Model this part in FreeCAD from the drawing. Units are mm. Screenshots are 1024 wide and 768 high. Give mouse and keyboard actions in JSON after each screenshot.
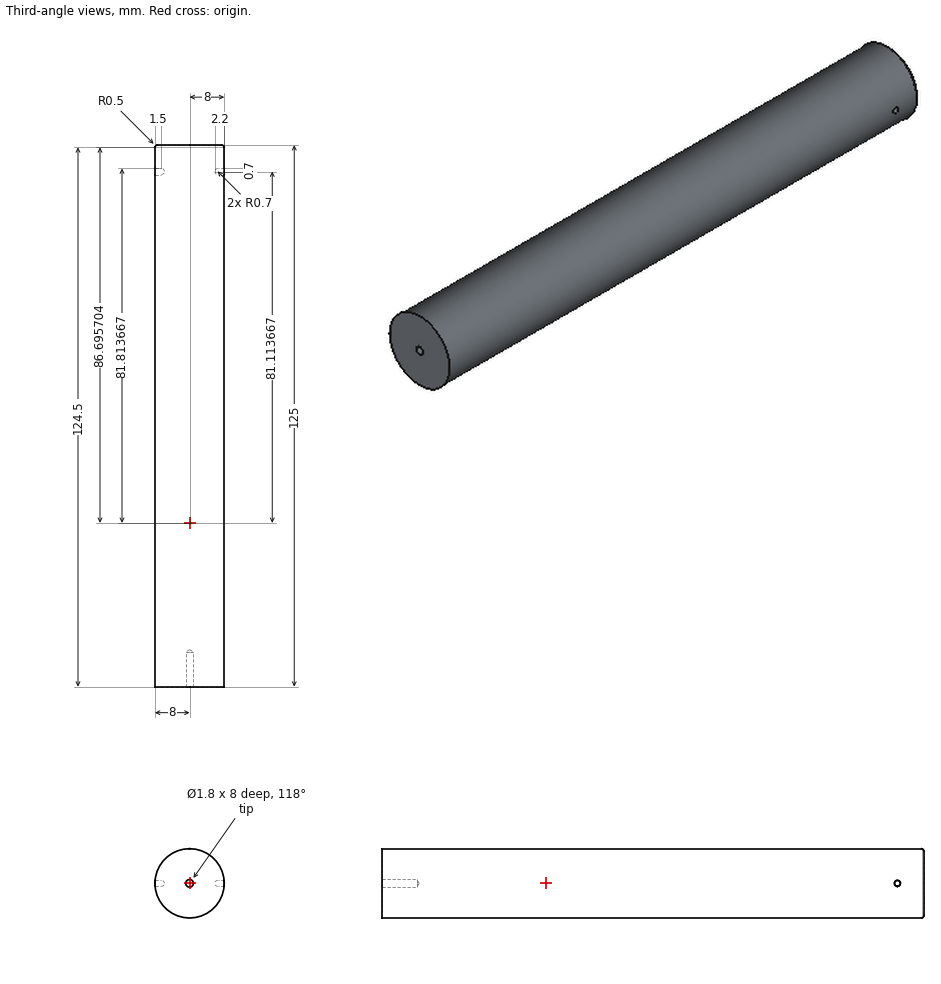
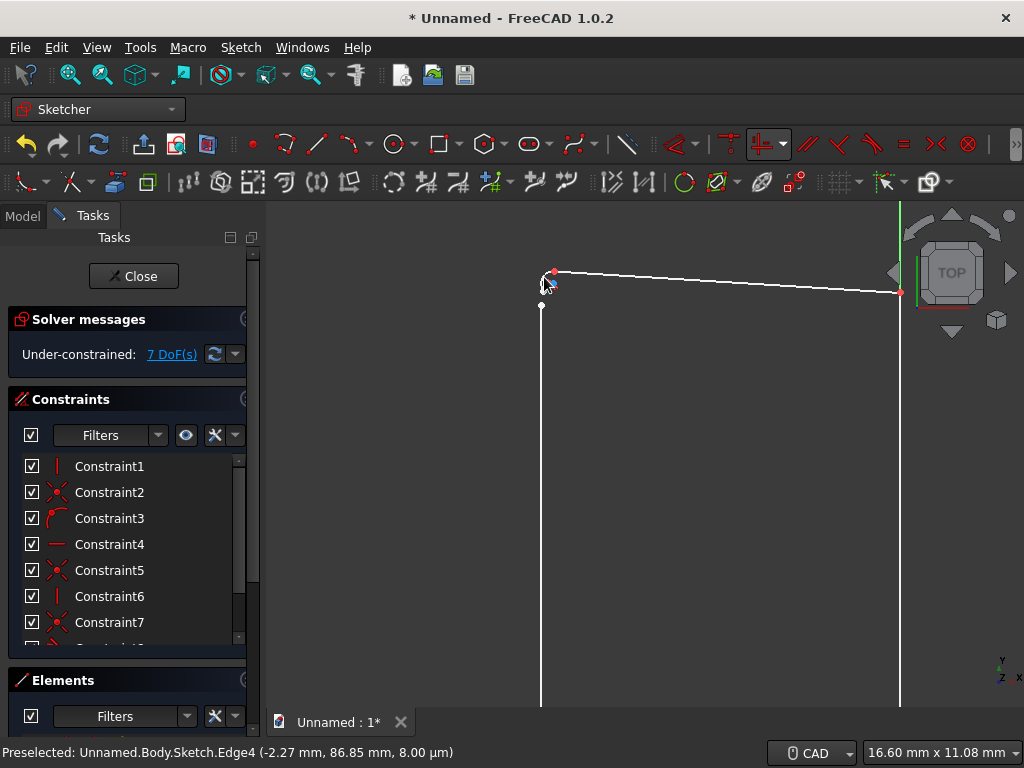
{"action": "scroll", "coordinate": [567, 281], "scroll_direction": "down", "scroll_amount": 14}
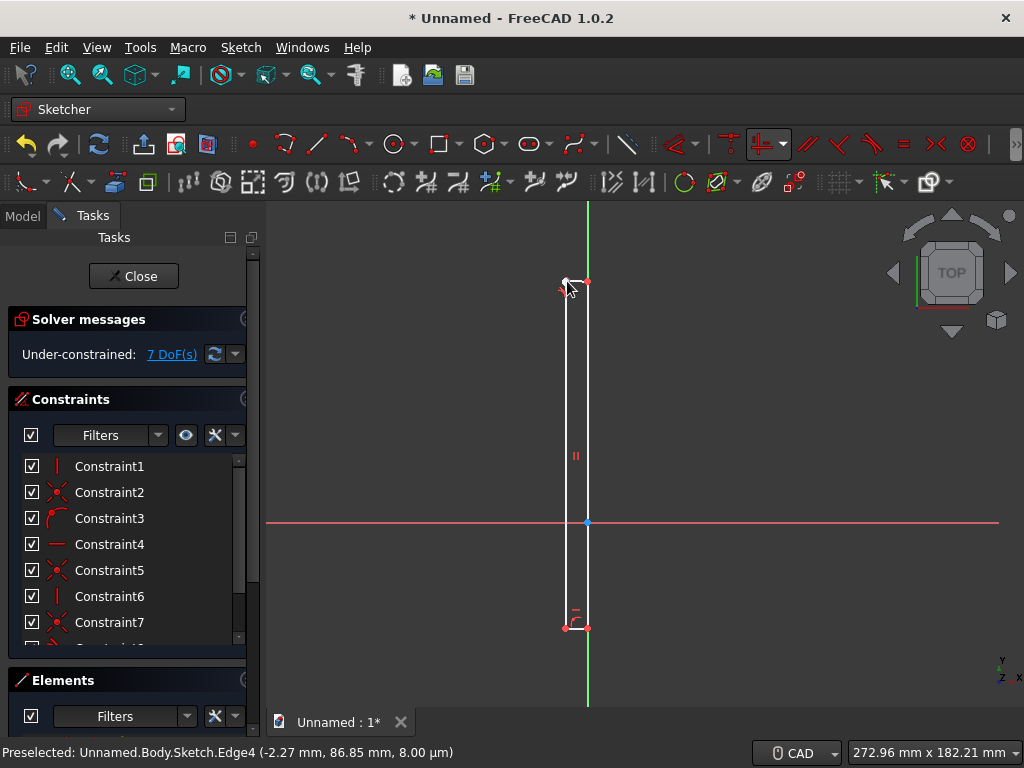
{"action": "scroll", "coordinate": [581, 281], "scroll_direction": "up", "scroll_amount": 4}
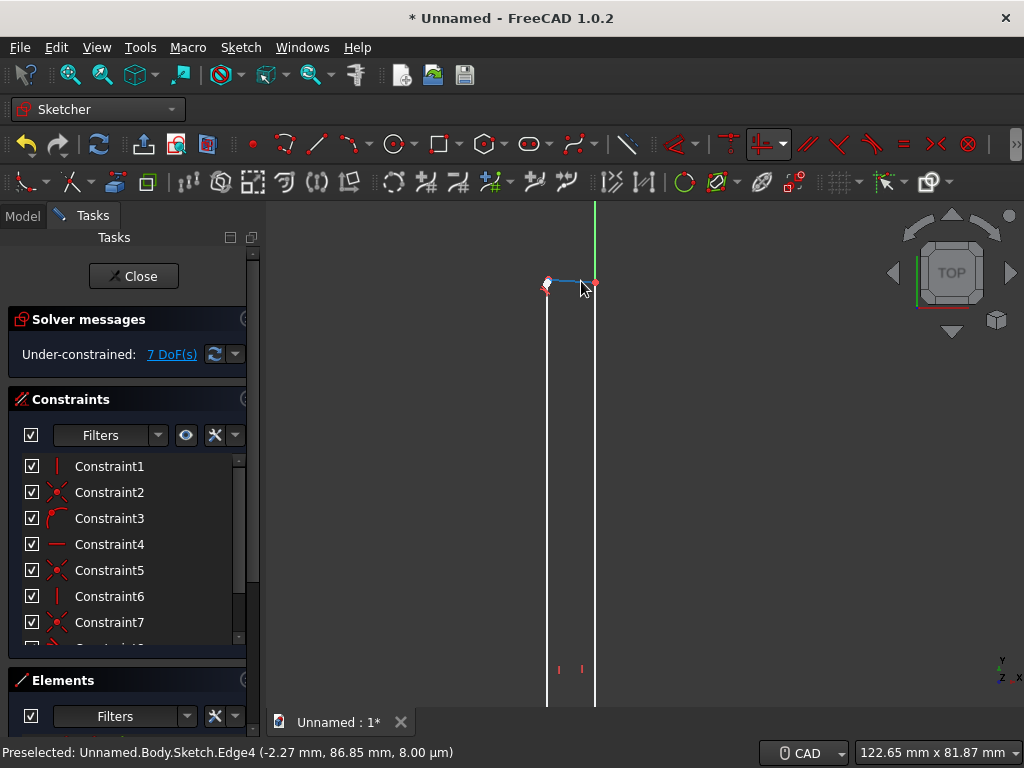
{"action": "left_click", "coordinate": [581, 282]}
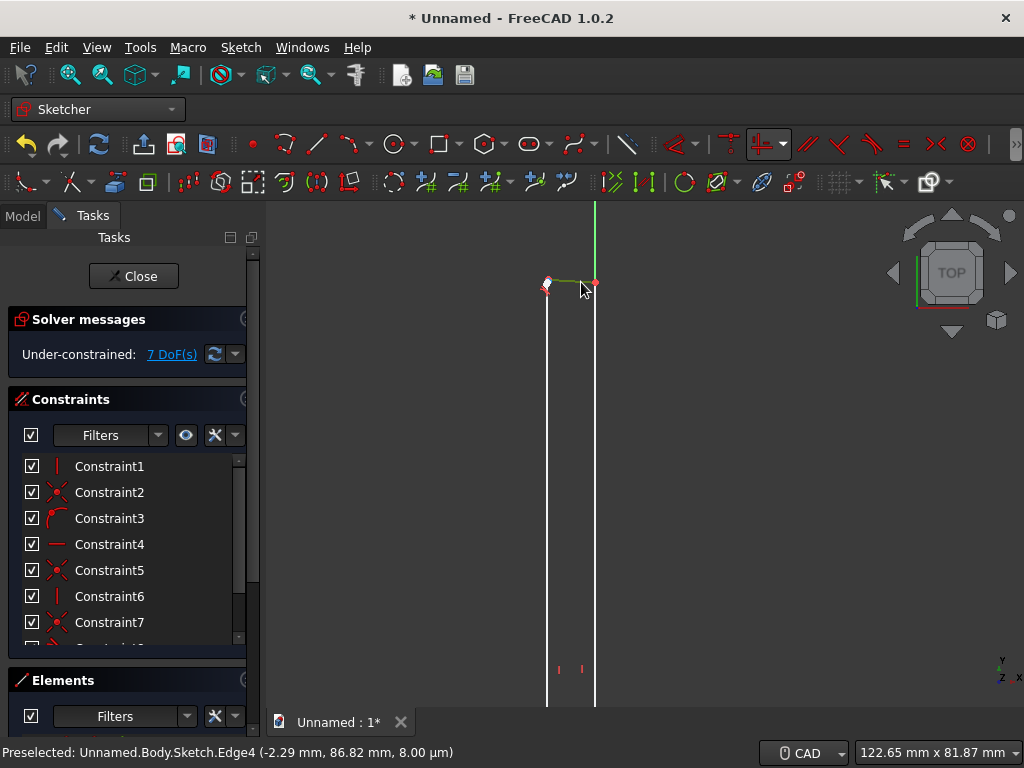
{"action": "left_click", "coordinate": [786, 144]}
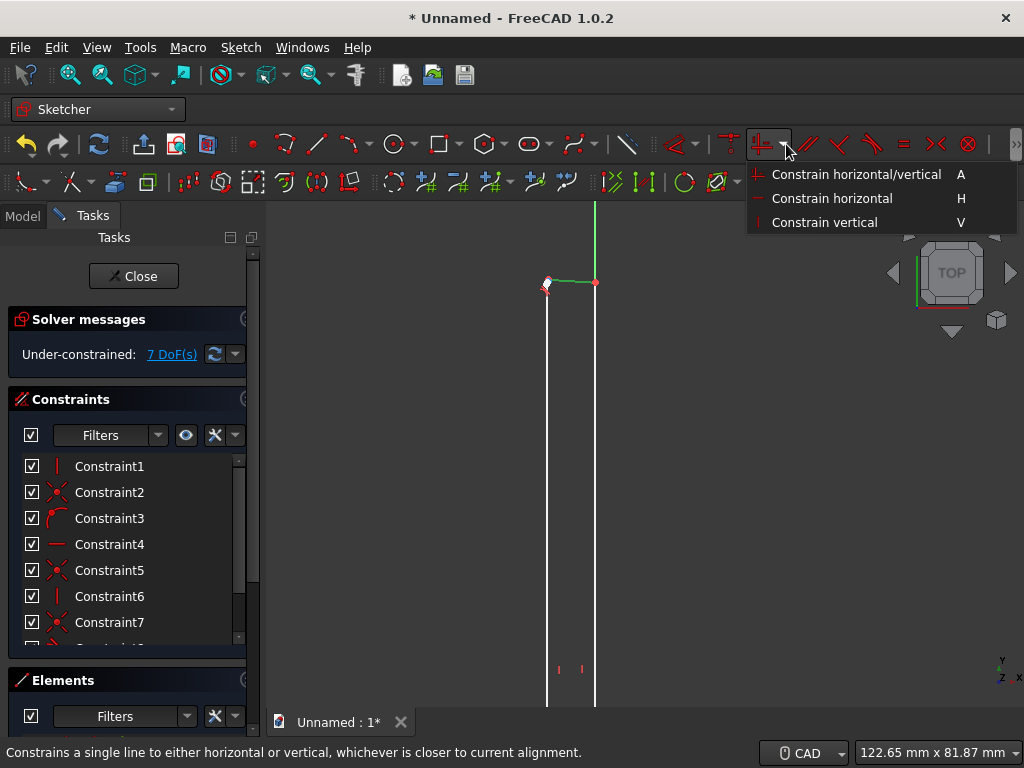
{"action": "left_click", "coordinate": [882, 198]}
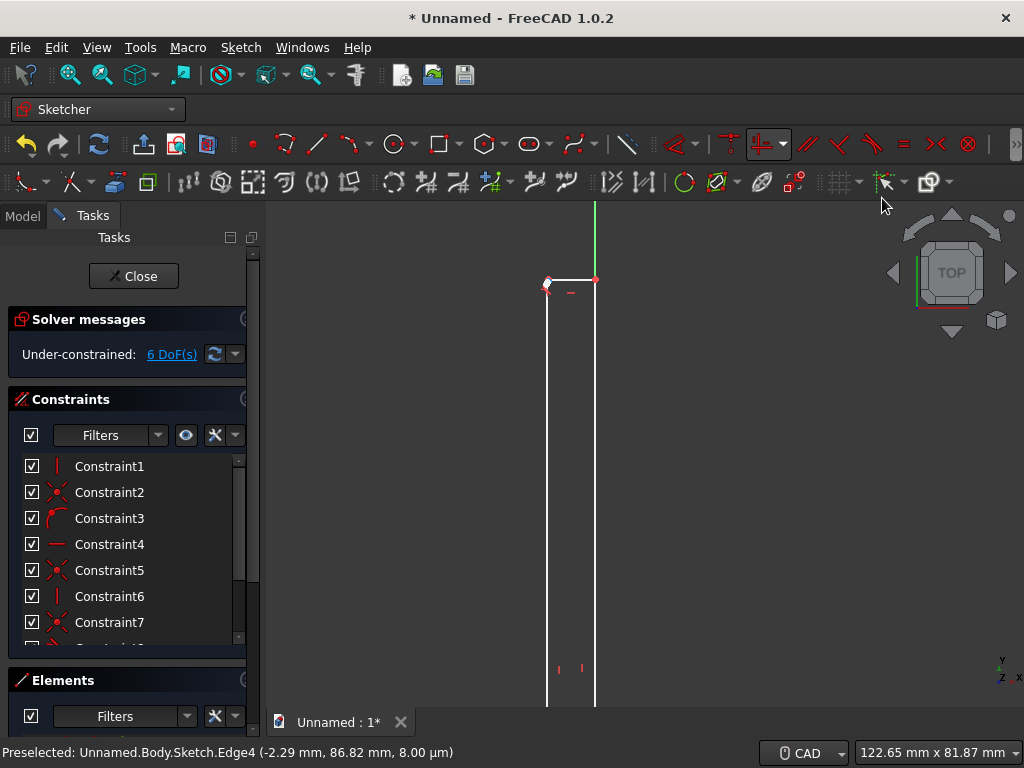
{"action": "scroll", "coordinate": [547, 281], "scroll_direction": "up", "scroll_amount": 13}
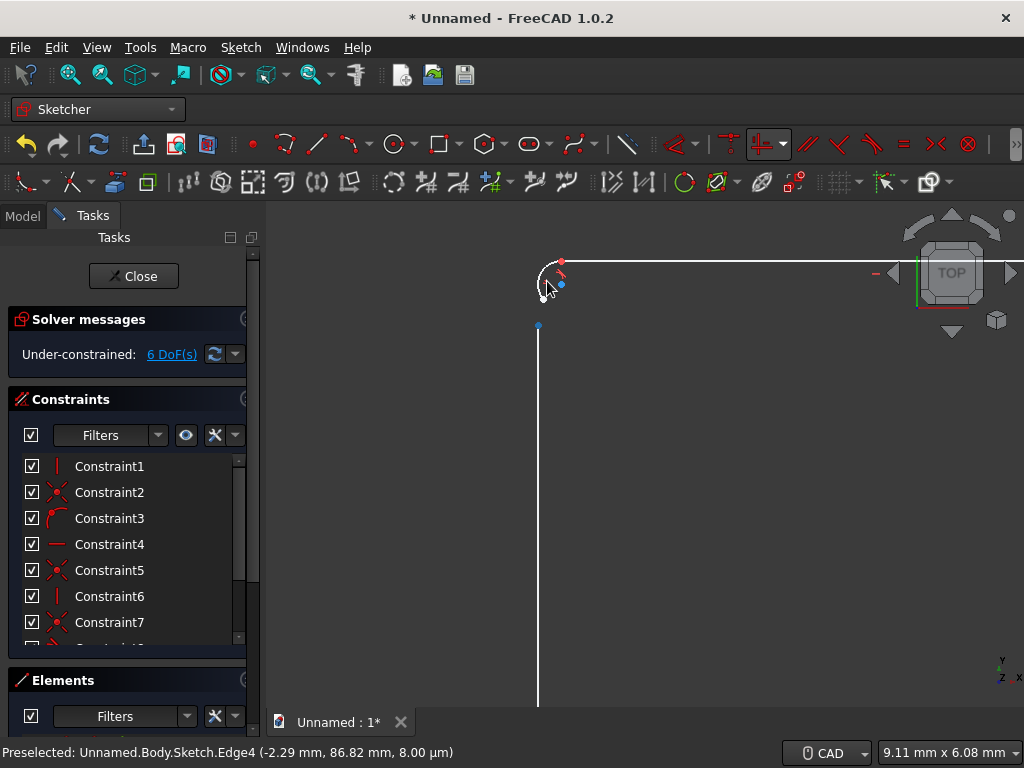
{"action": "left_click", "coordinate": [540, 274]}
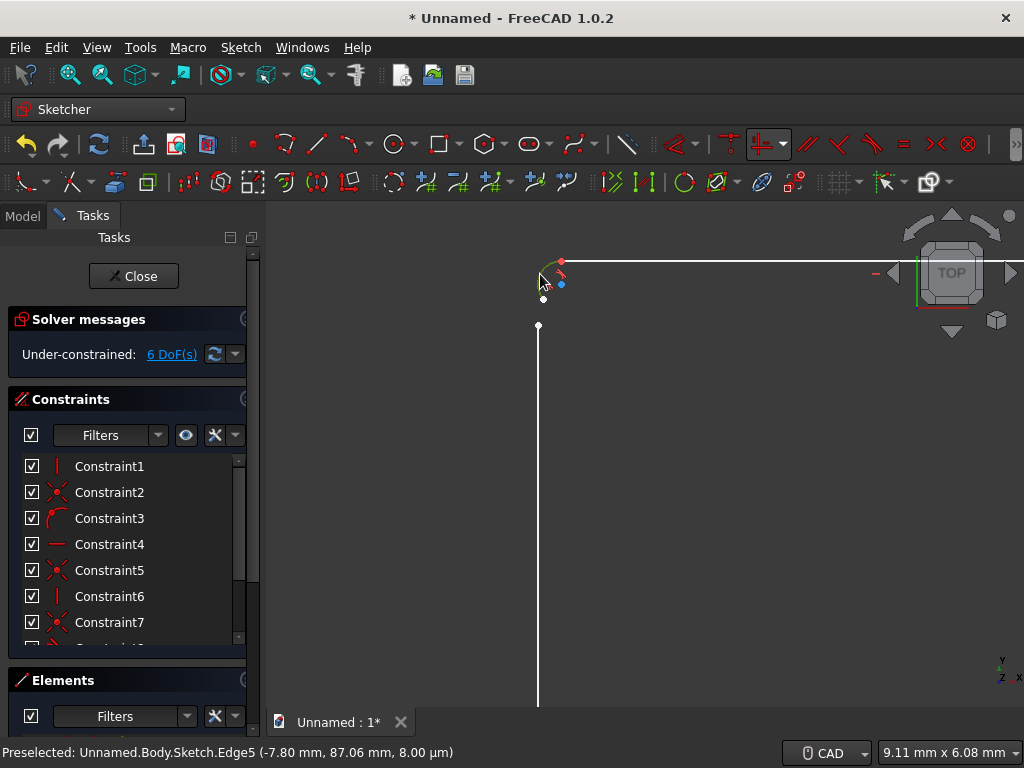
{"action": "key", "text": "k r"}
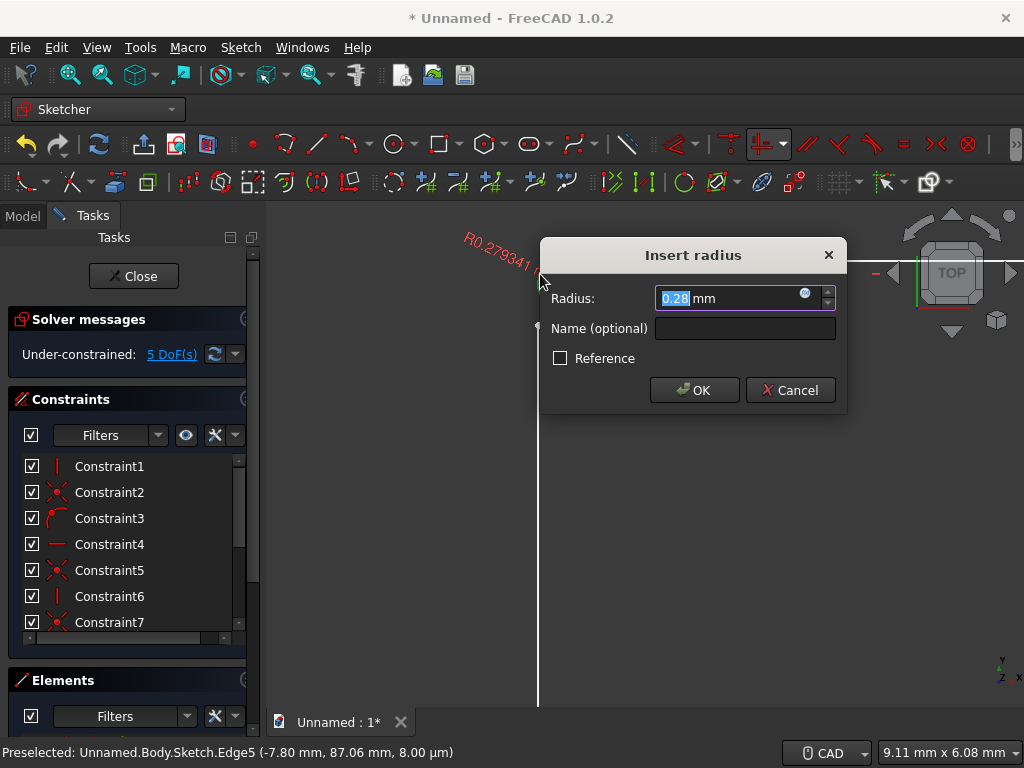
{"action": "type", "text": "0.5"}
{"action": "key", "text": "Return"}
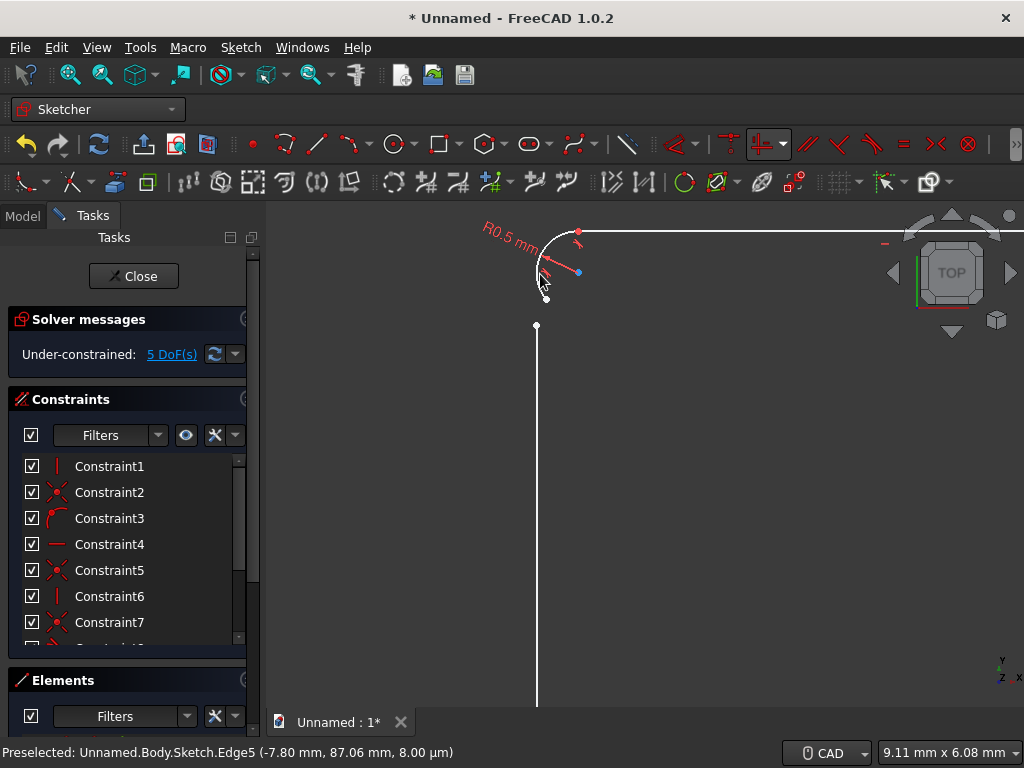
{"action": "scroll", "coordinate": [567, 281], "scroll_direction": "down", "scroll_amount": 17}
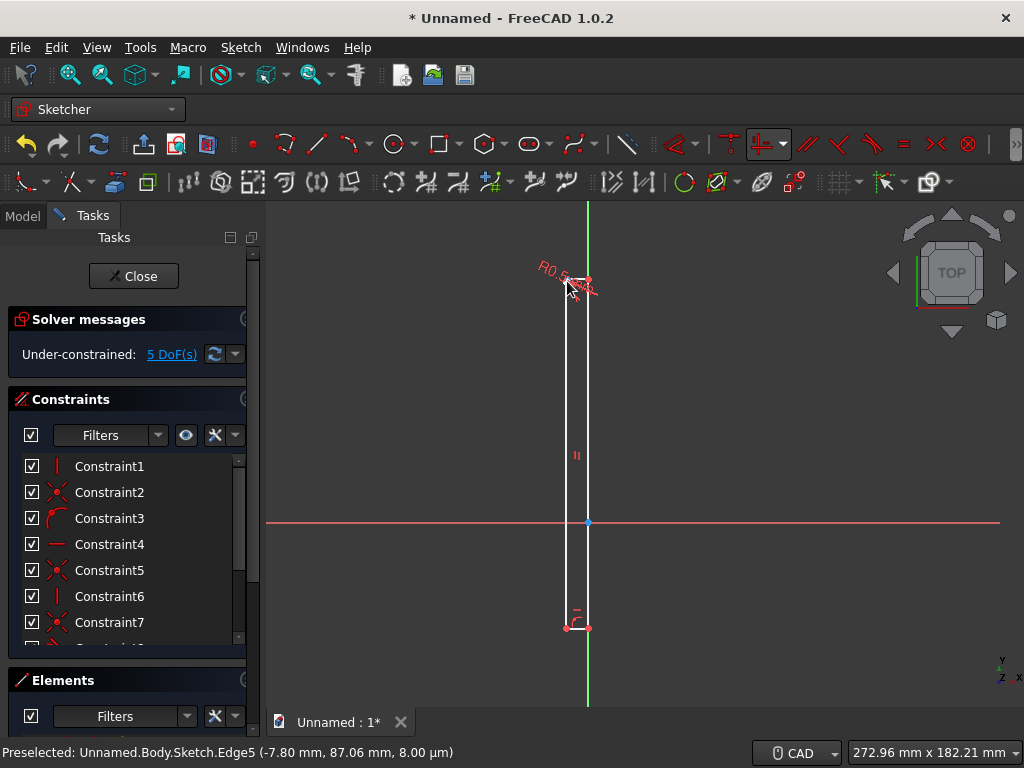
{"action": "scroll", "coordinate": [573, 629], "scroll_direction": "up", "scroll_amount": 4}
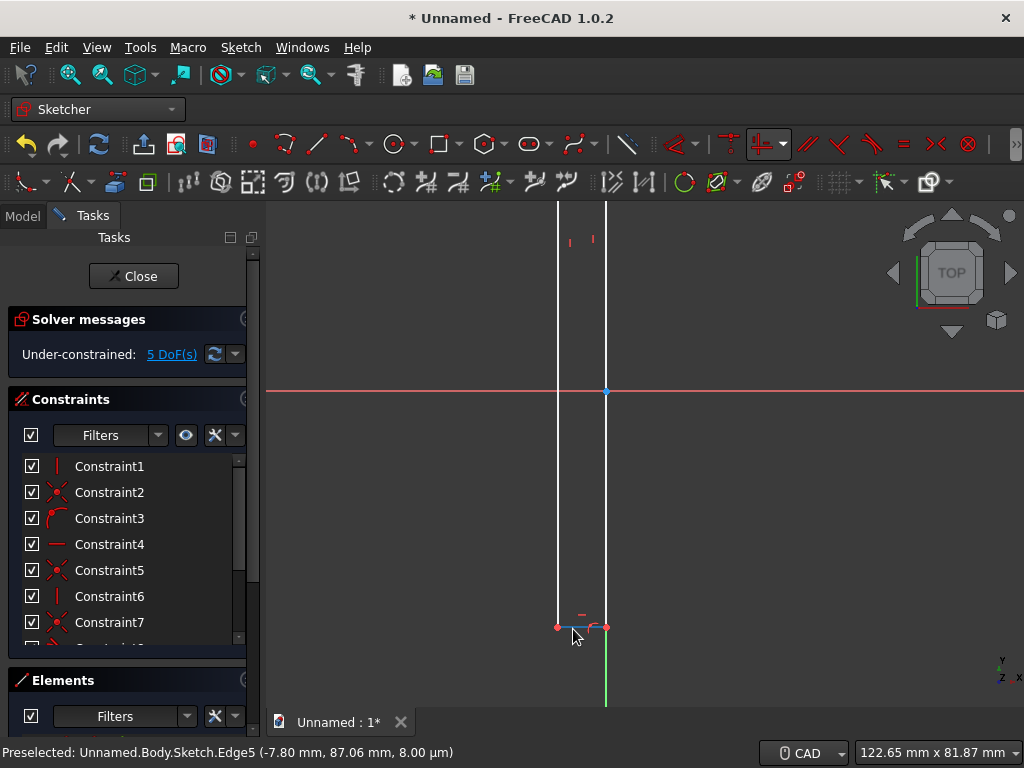
{"action": "left_click", "coordinate": [572, 627]}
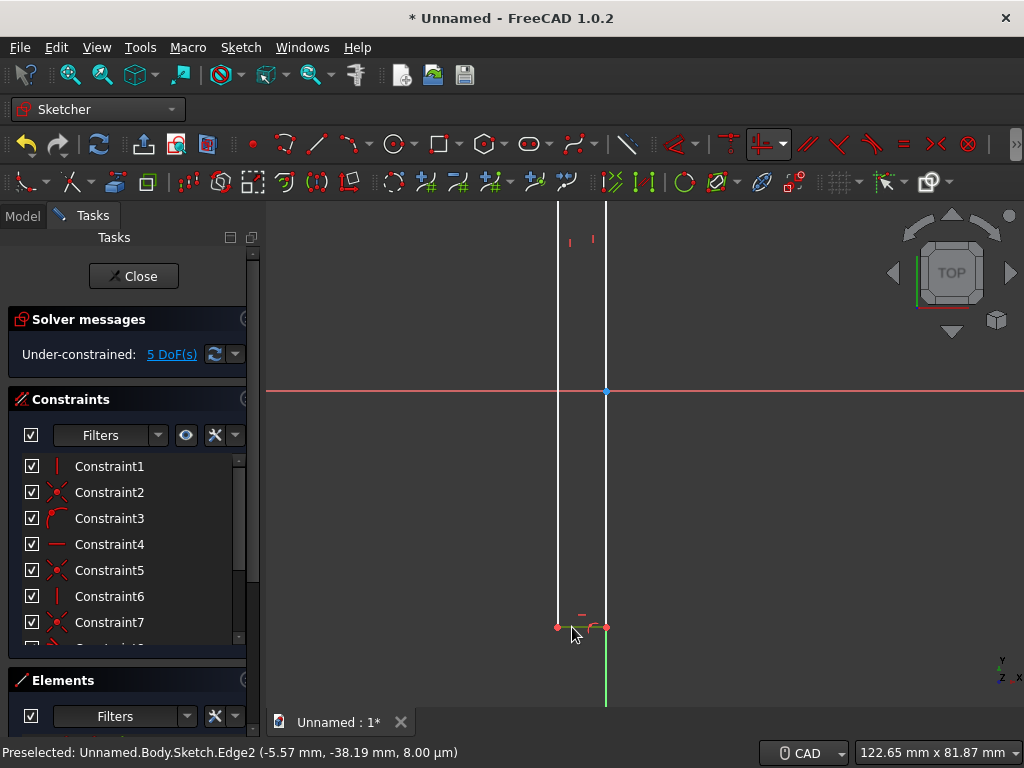
{"action": "key", "text": "l"}